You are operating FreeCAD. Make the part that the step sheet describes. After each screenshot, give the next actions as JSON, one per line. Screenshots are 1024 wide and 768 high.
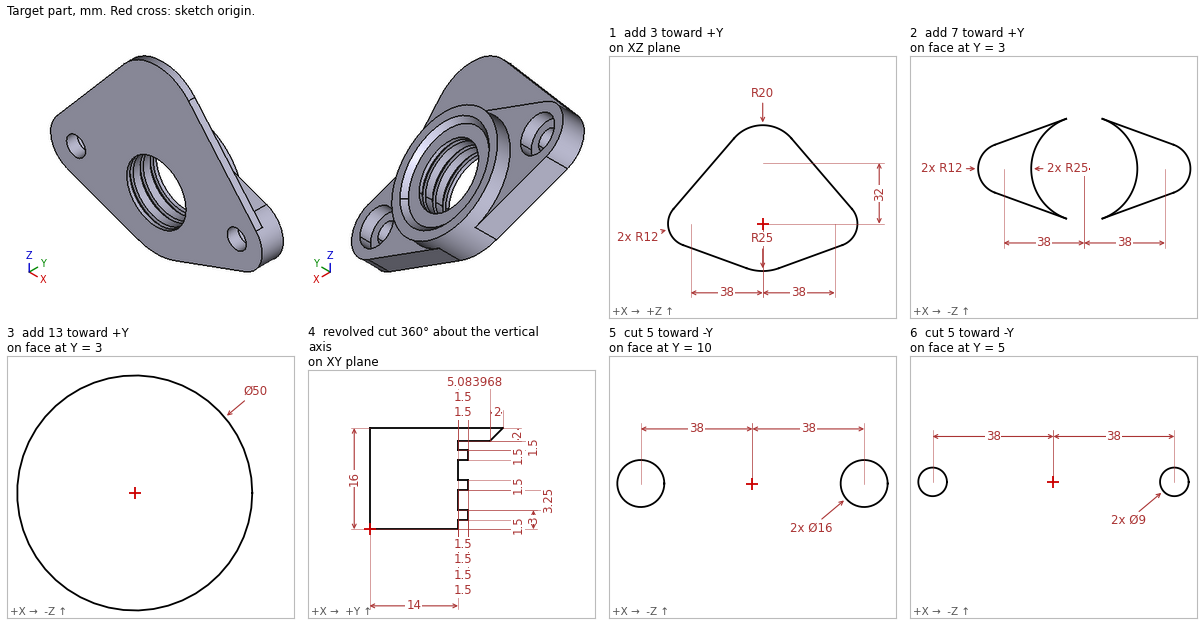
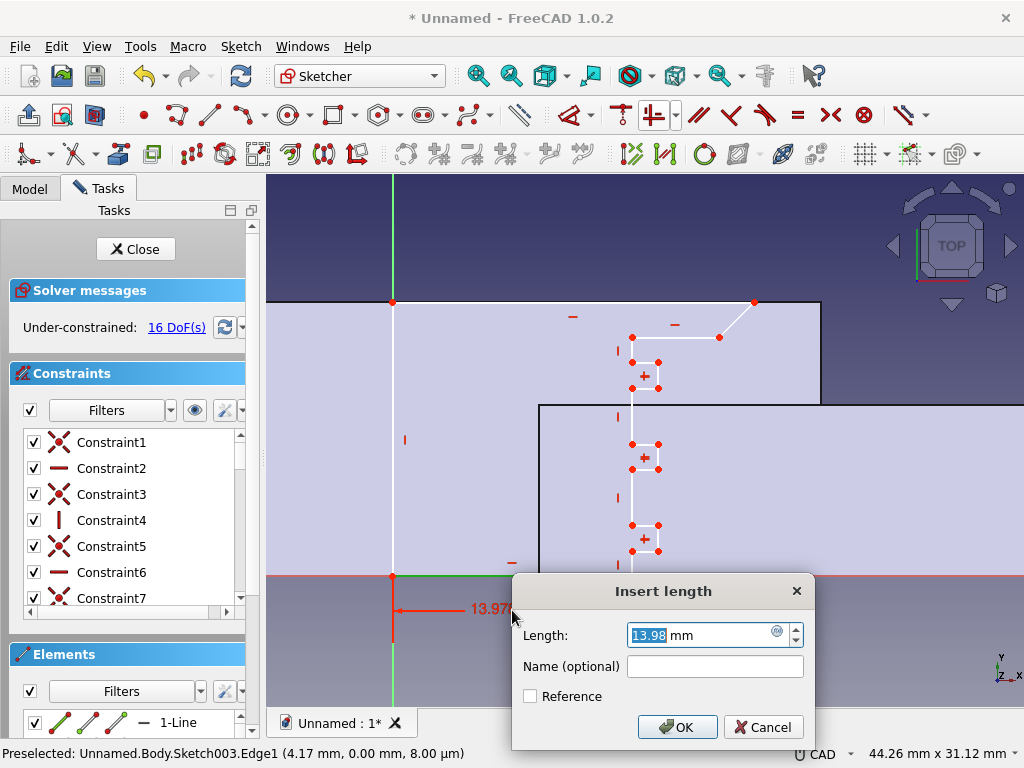
{"action": "type", "text": "14"}
{"action": "key", "text": "Return"}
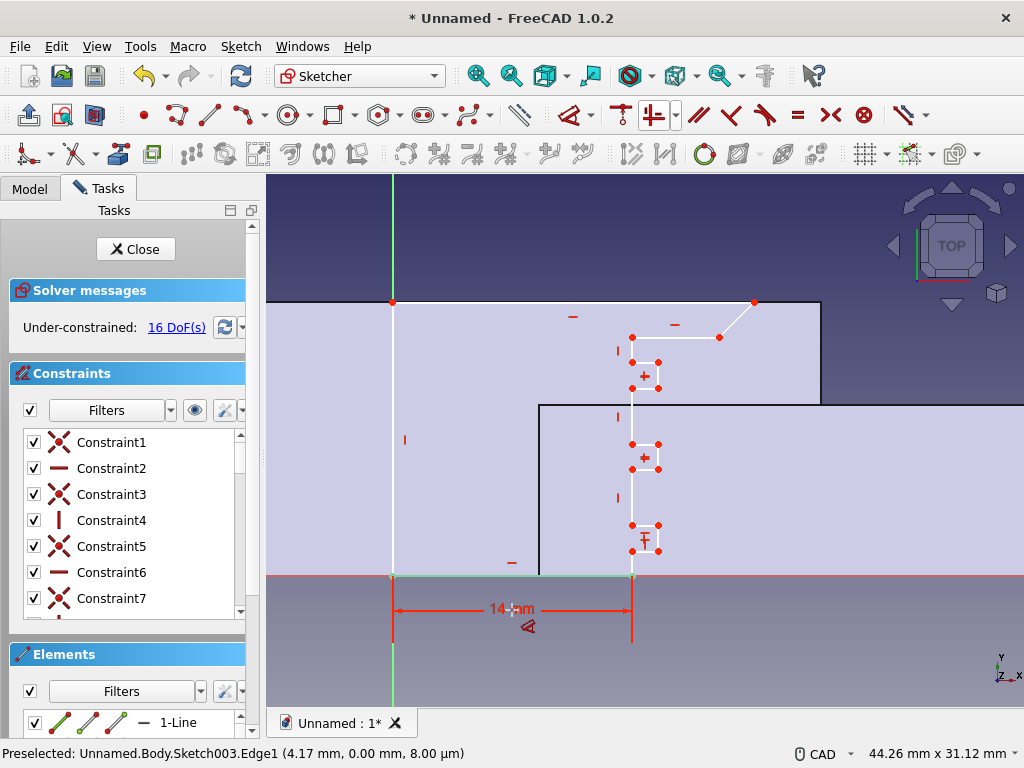
{"action": "left_click", "coordinate": [393, 385]}
{"action": "left_click", "coordinate": [359, 440]}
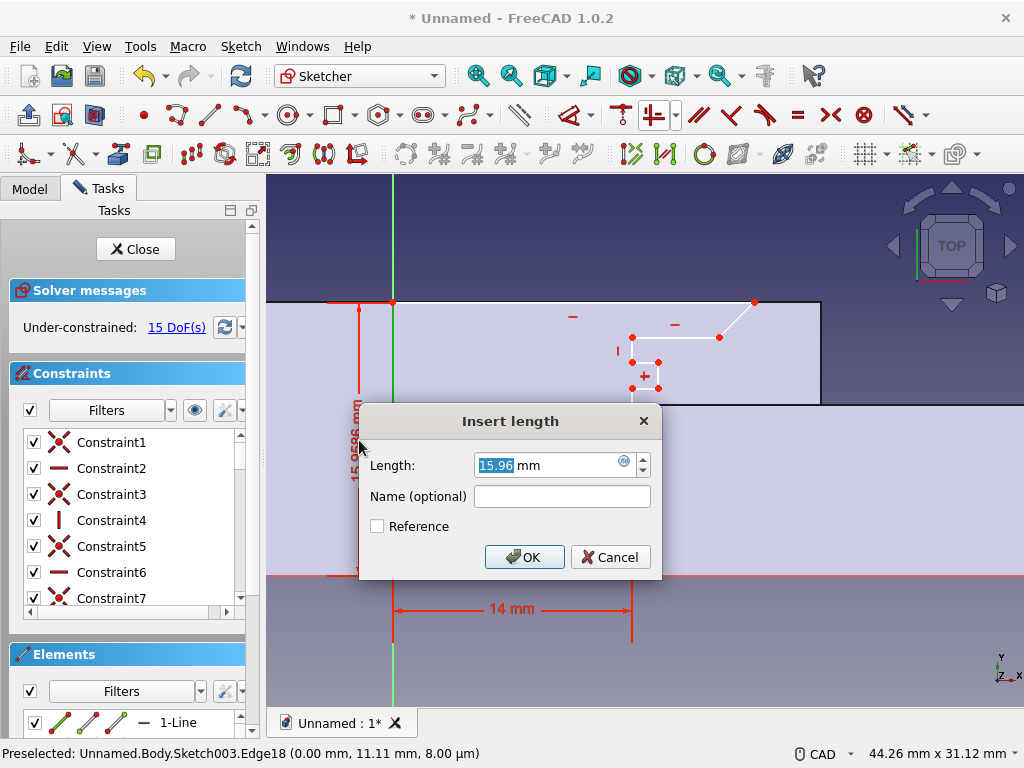
{"action": "type", "text": "16"}
{"action": "key", "text": "Return"}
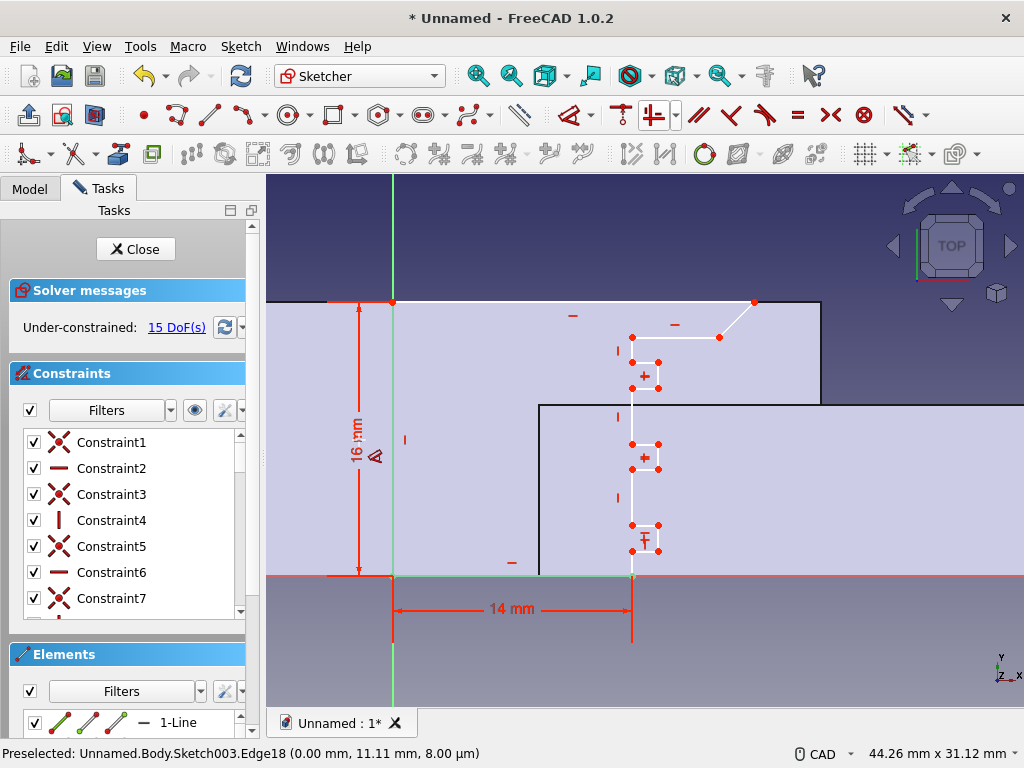
{"action": "left_click", "coordinate": [658, 526]}
{"action": "left_click", "coordinate": [359, 551]}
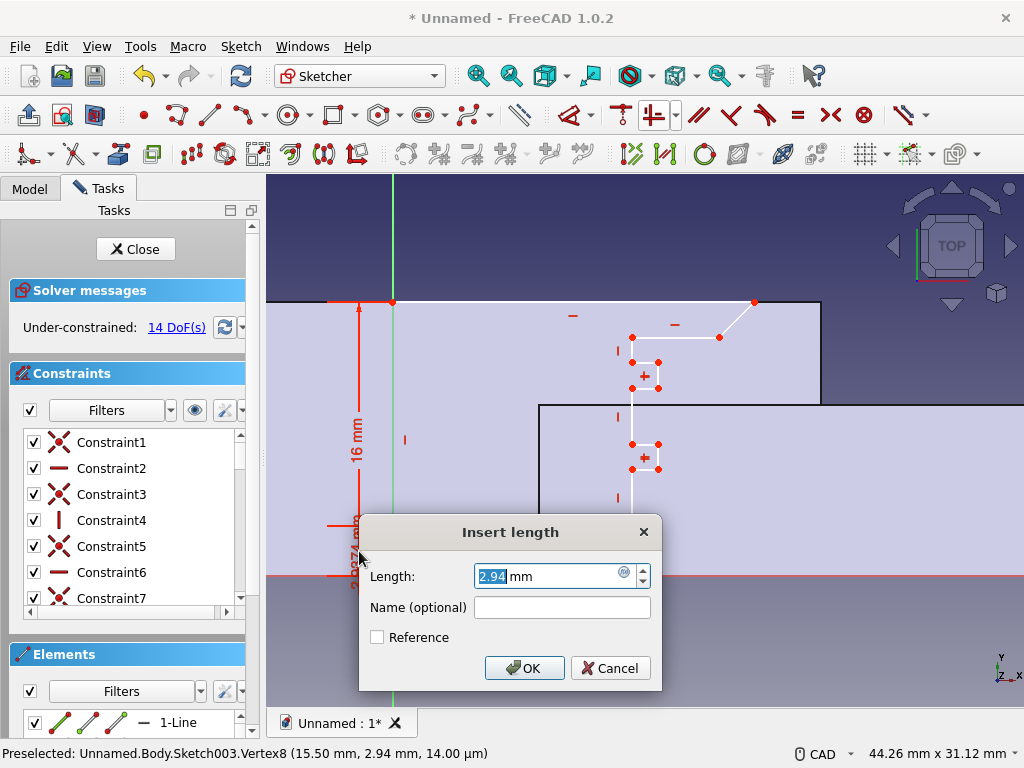
{"action": "type", "text": "3"}
{"action": "key", "text": "Return"}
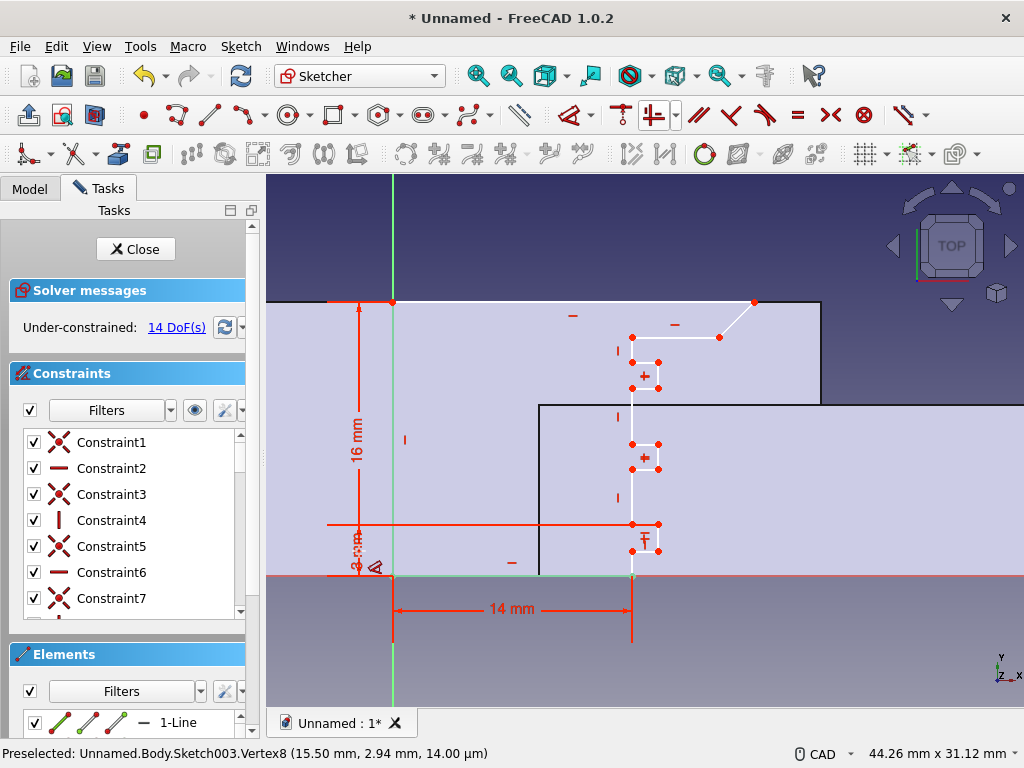
{"action": "left_click", "coordinate": [729, 327]}
{"action": "left_click", "coordinate": [736, 268]}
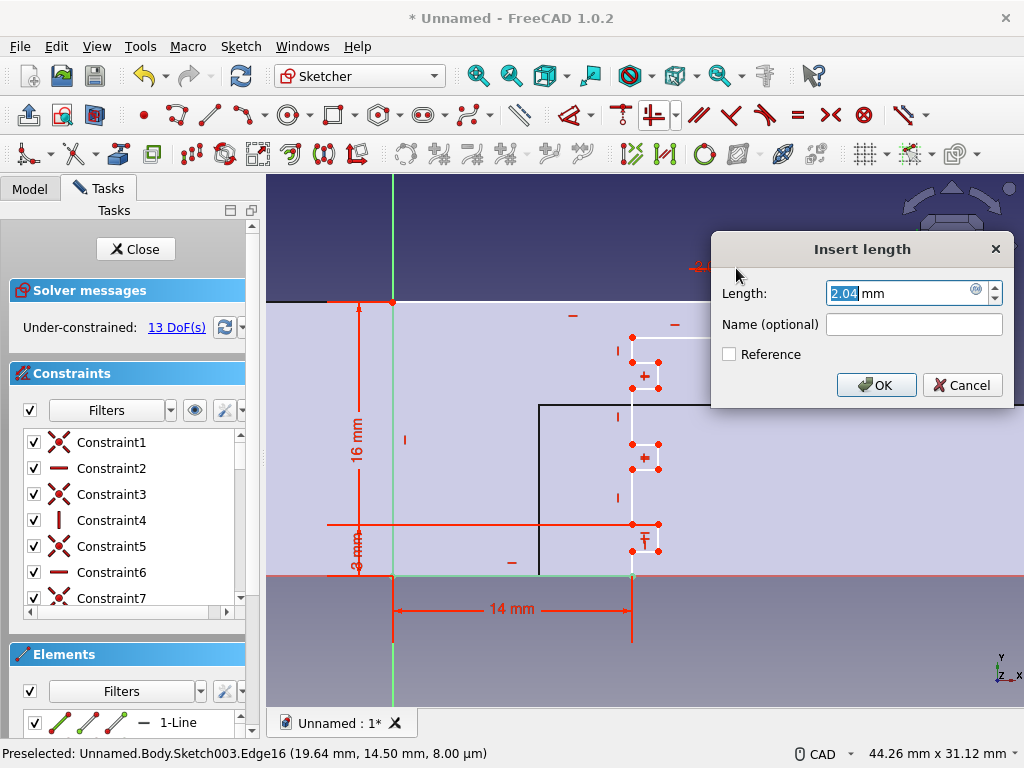
{"action": "type", "text": "2"}
{"action": "key", "text": "Return"}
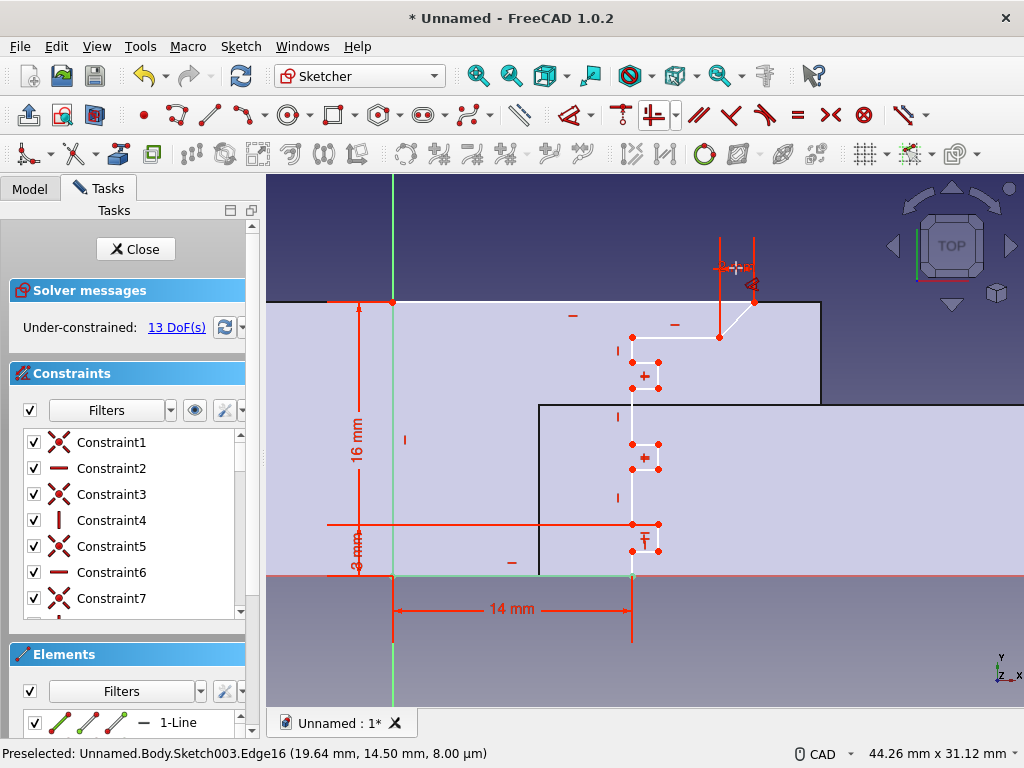
{"action": "left_click", "coordinate": [730, 327]}
{"action": "left_click", "coordinate": [788, 320]}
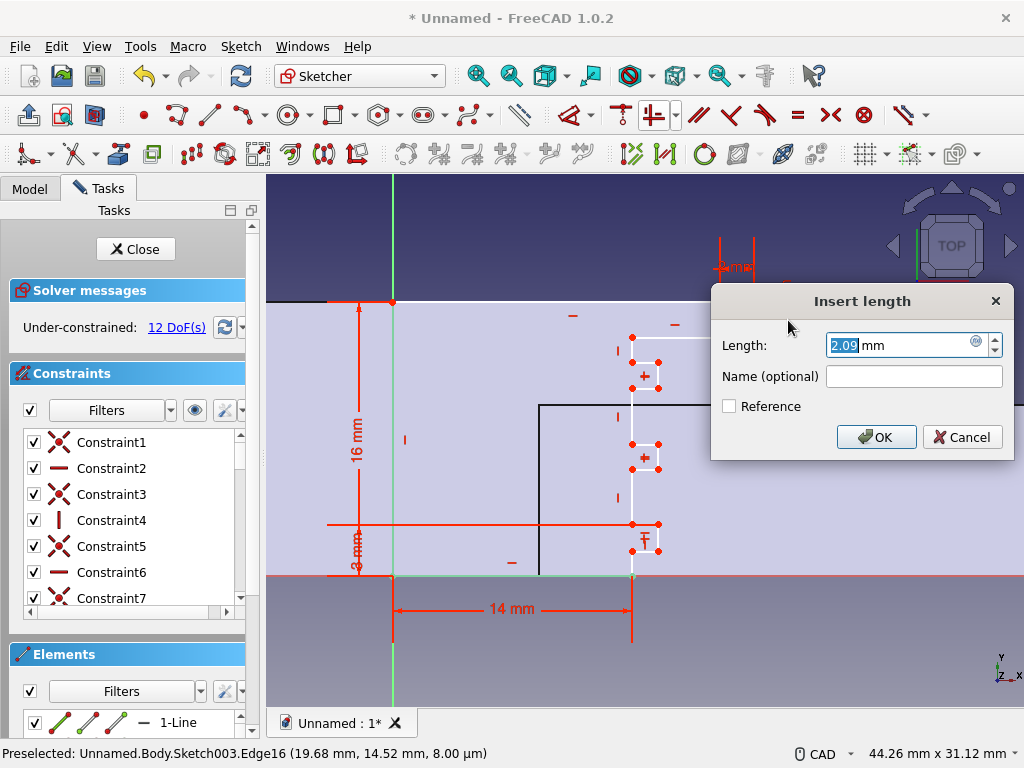
{"action": "type", "text": "2"}
{"action": "key", "text": "Return"}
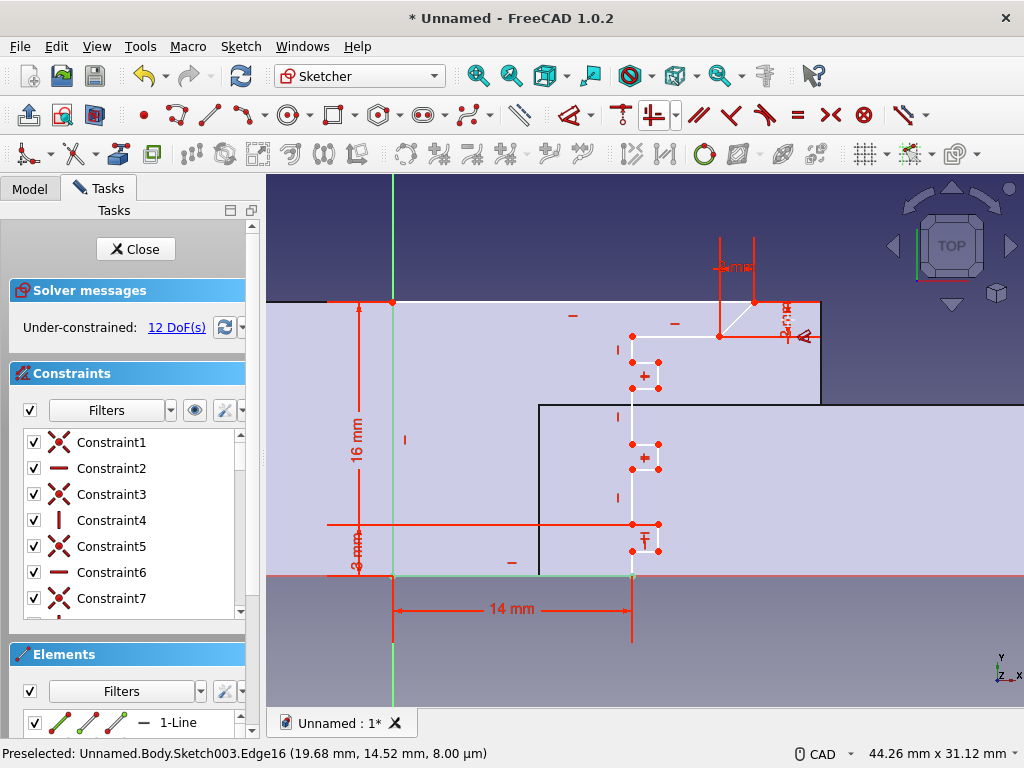
{"action": "scroll", "coordinate": [632, 567], "scroll_direction": "up", "scroll_amount": 3}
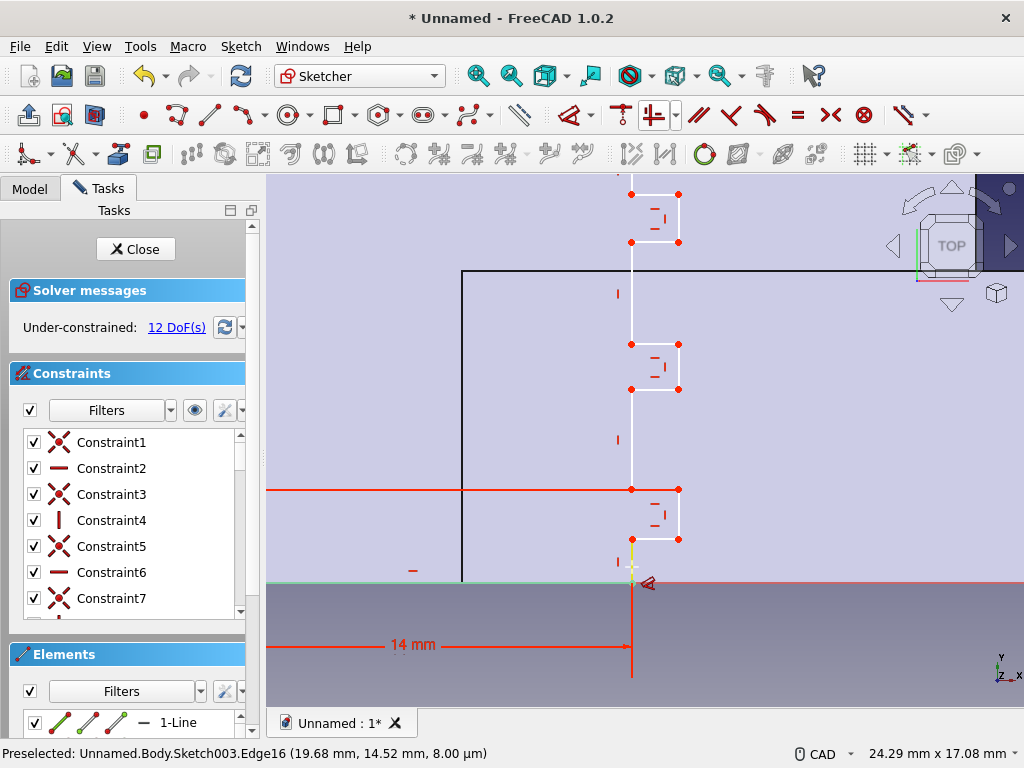
{"action": "left_click", "coordinate": [632, 566]}
{"action": "left_click", "coordinate": [666, 561]}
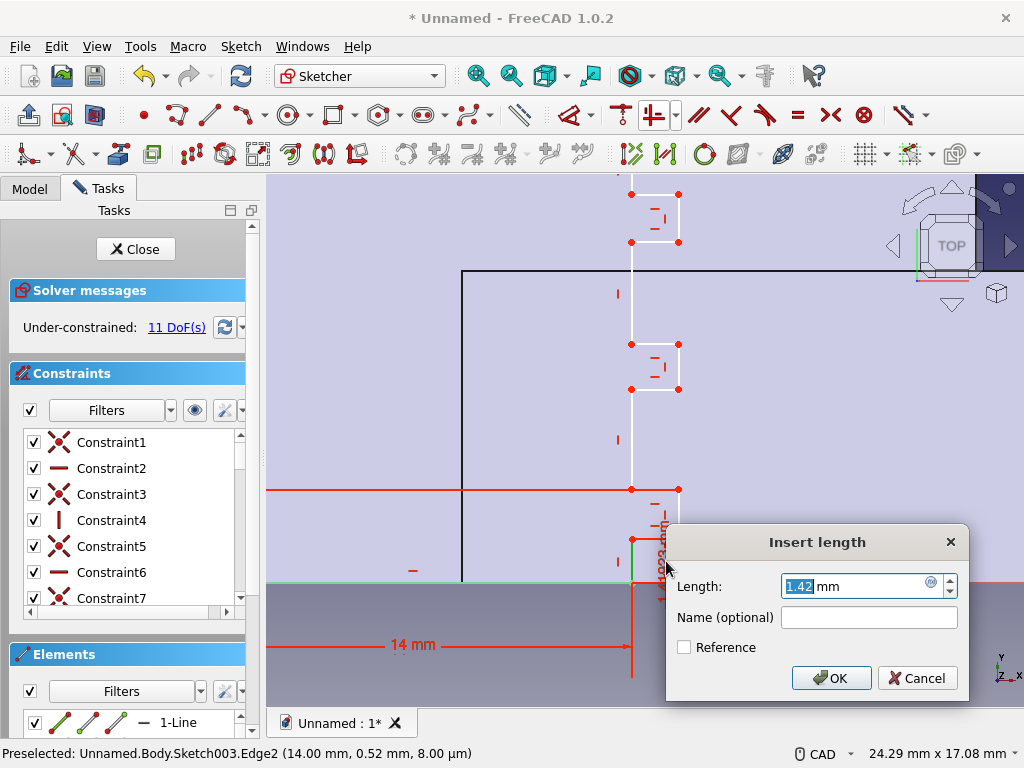
{"action": "type", "text": "1.5"}
{"action": "key", "text": "Return"}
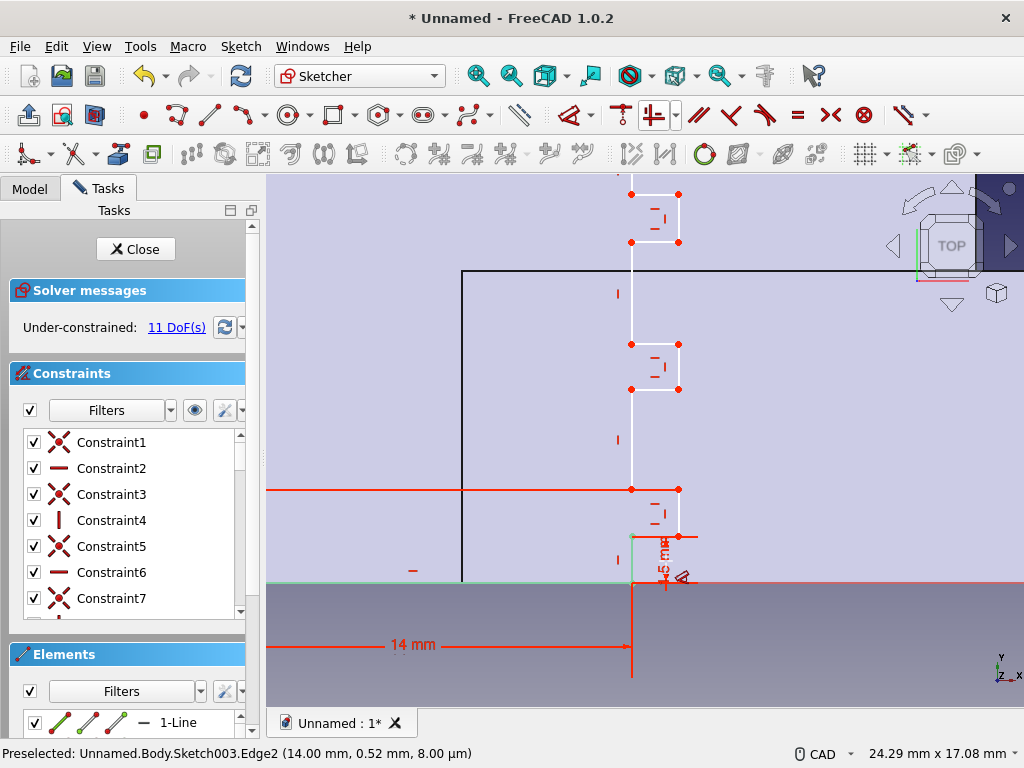
{"action": "left_click", "coordinate": [646, 537]}
{"action": "left_click", "coordinate": [656, 619]}